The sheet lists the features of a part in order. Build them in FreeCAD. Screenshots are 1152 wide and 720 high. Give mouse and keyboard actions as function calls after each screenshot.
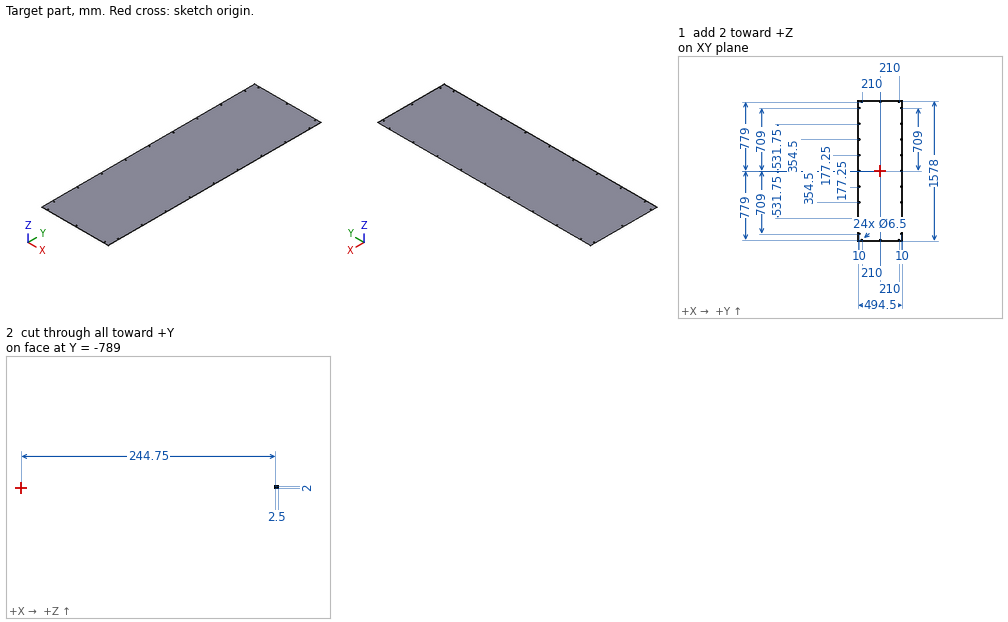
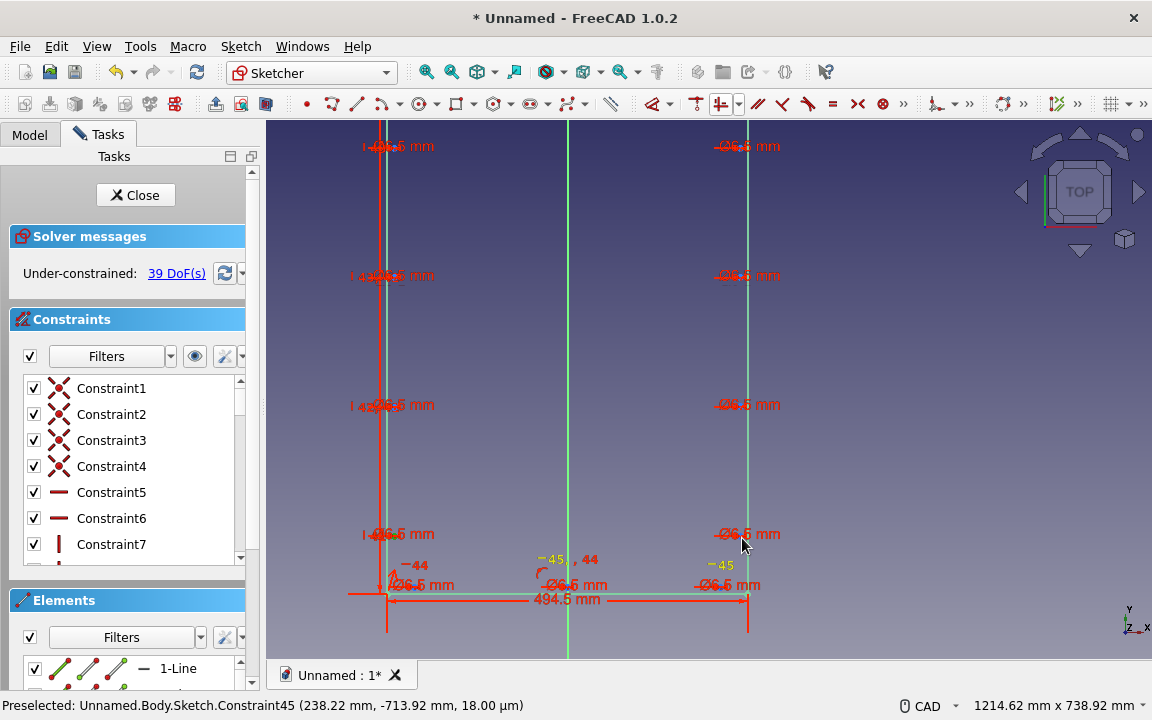
click(741, 536)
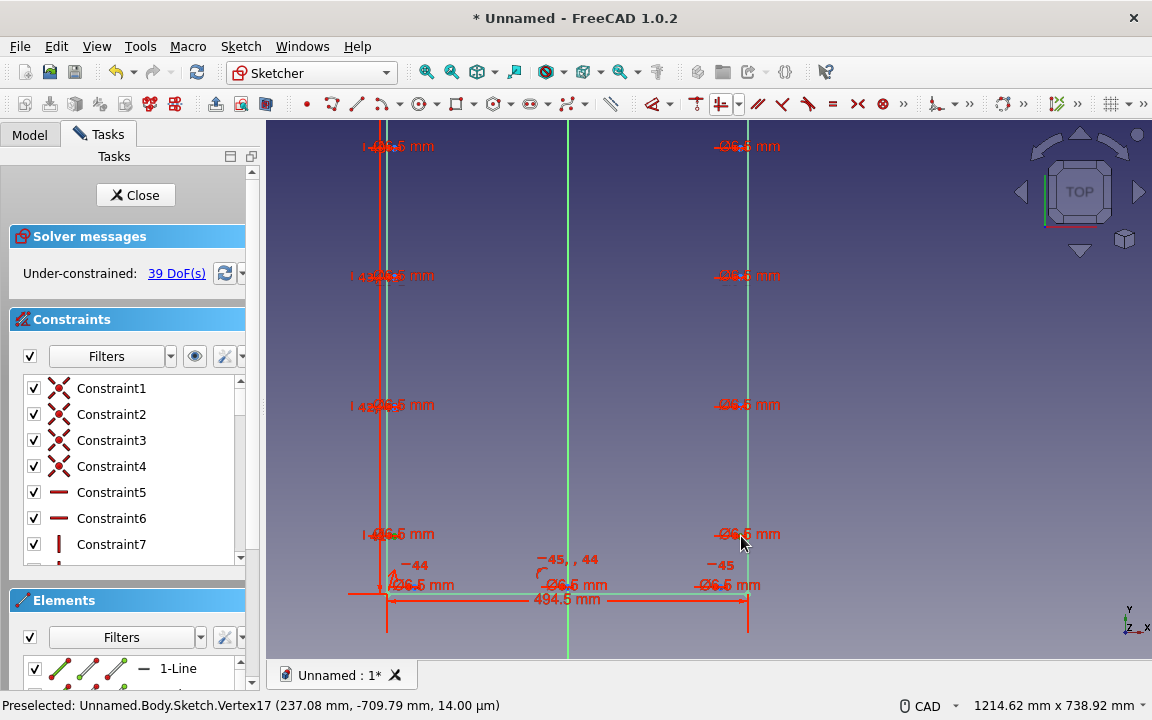
click(738, 104)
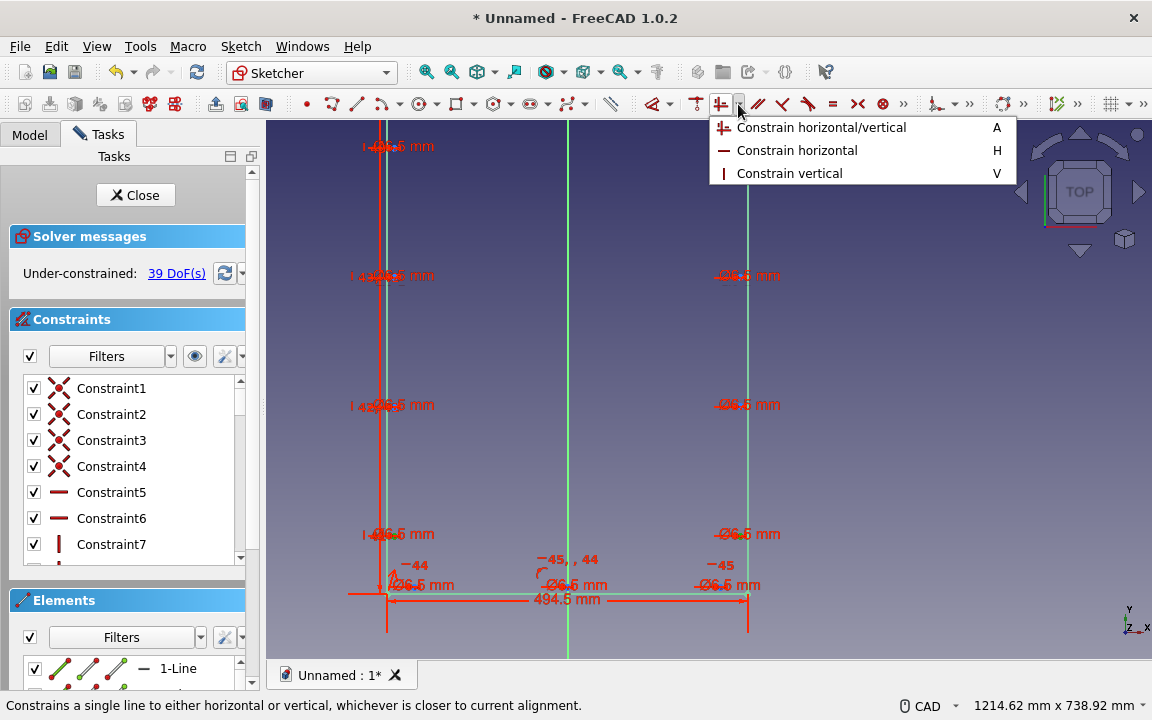
click(863, 150)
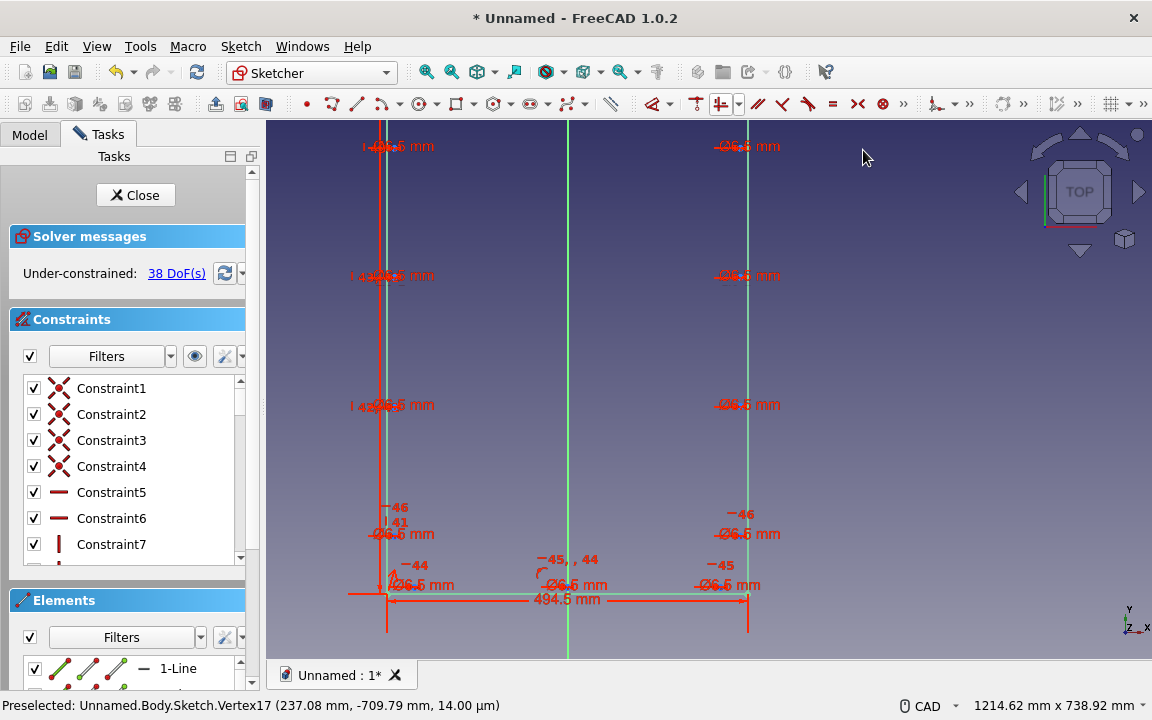
click(741, 536)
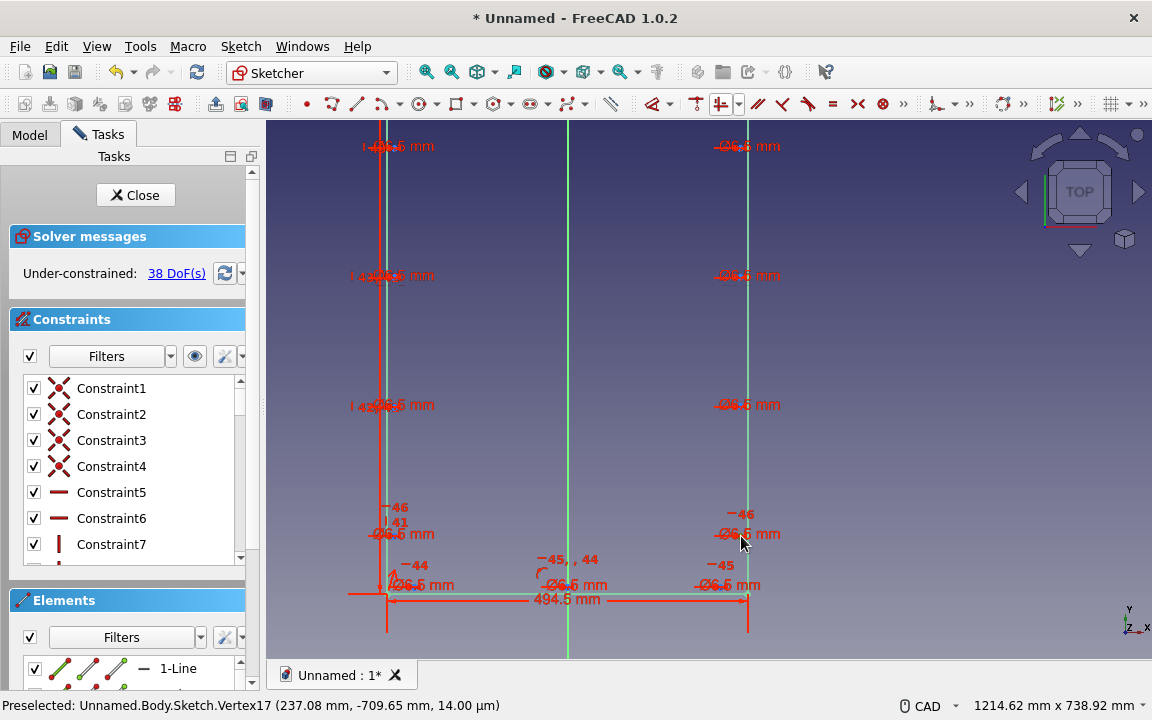
click(740, 407)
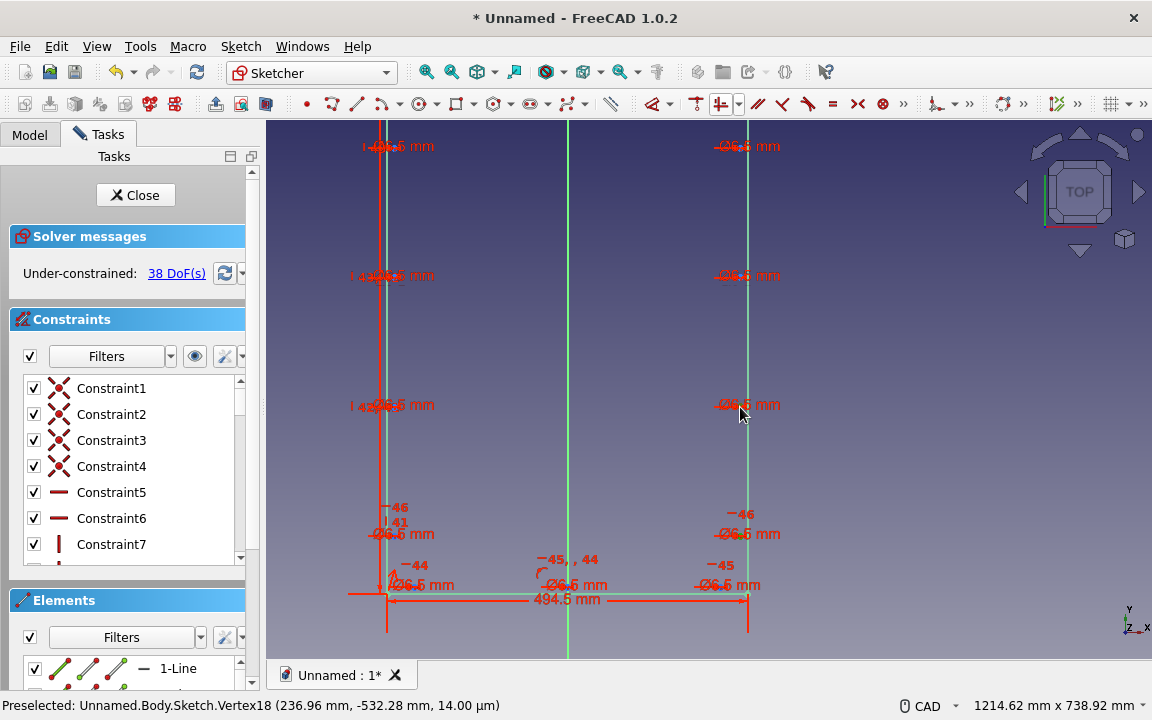
click(738, 104)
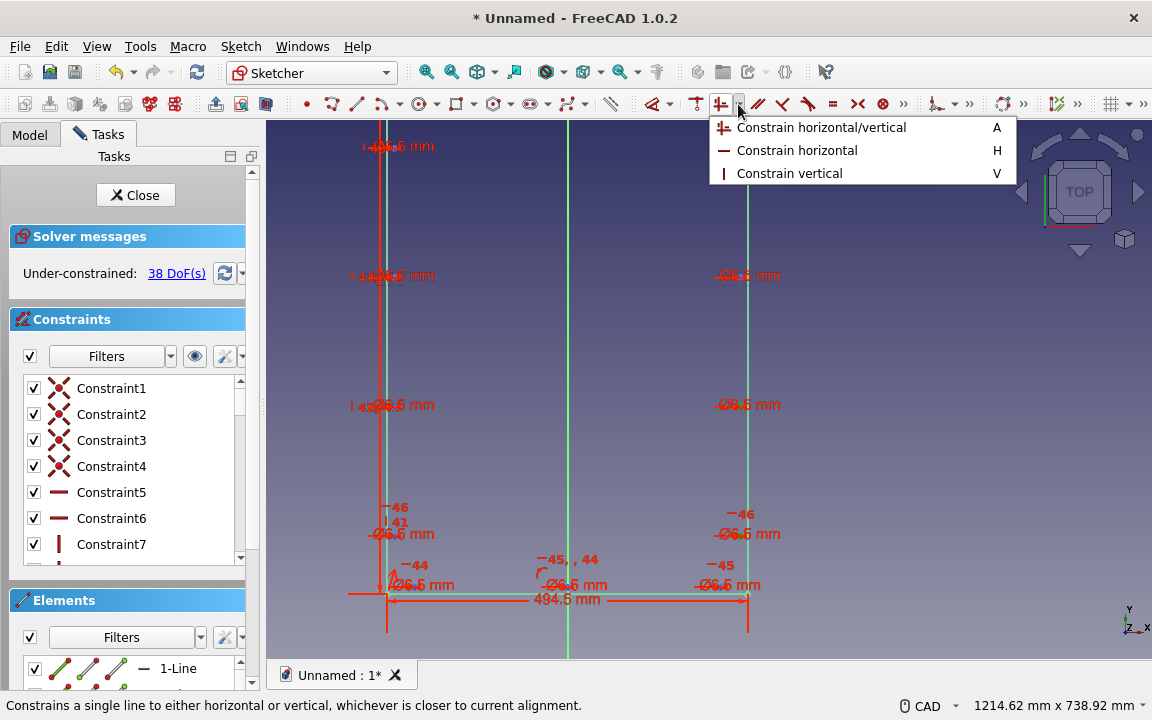
click(863, 174)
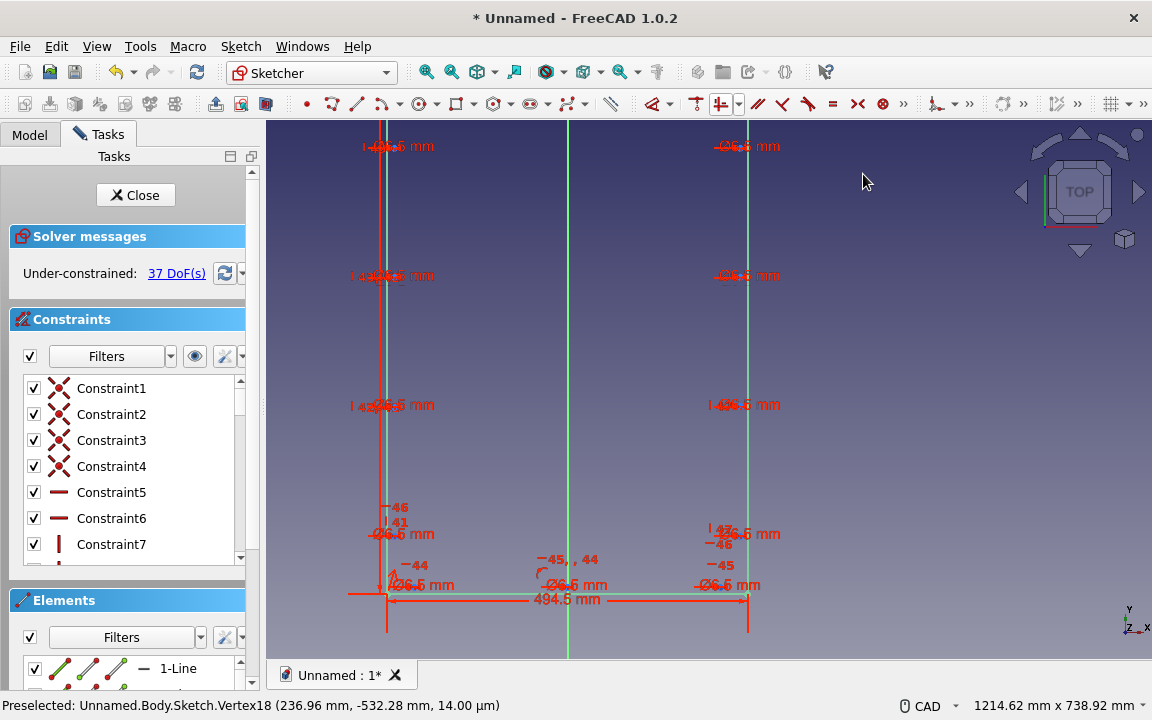
click(394, 407)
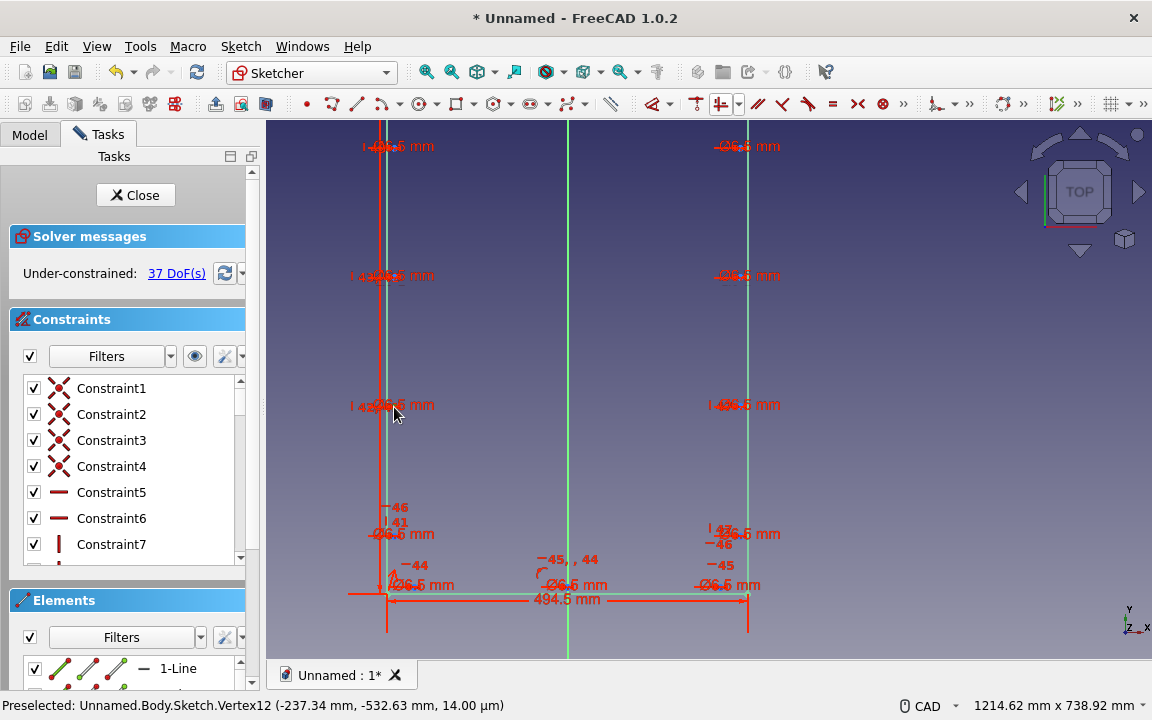
click(741, 407)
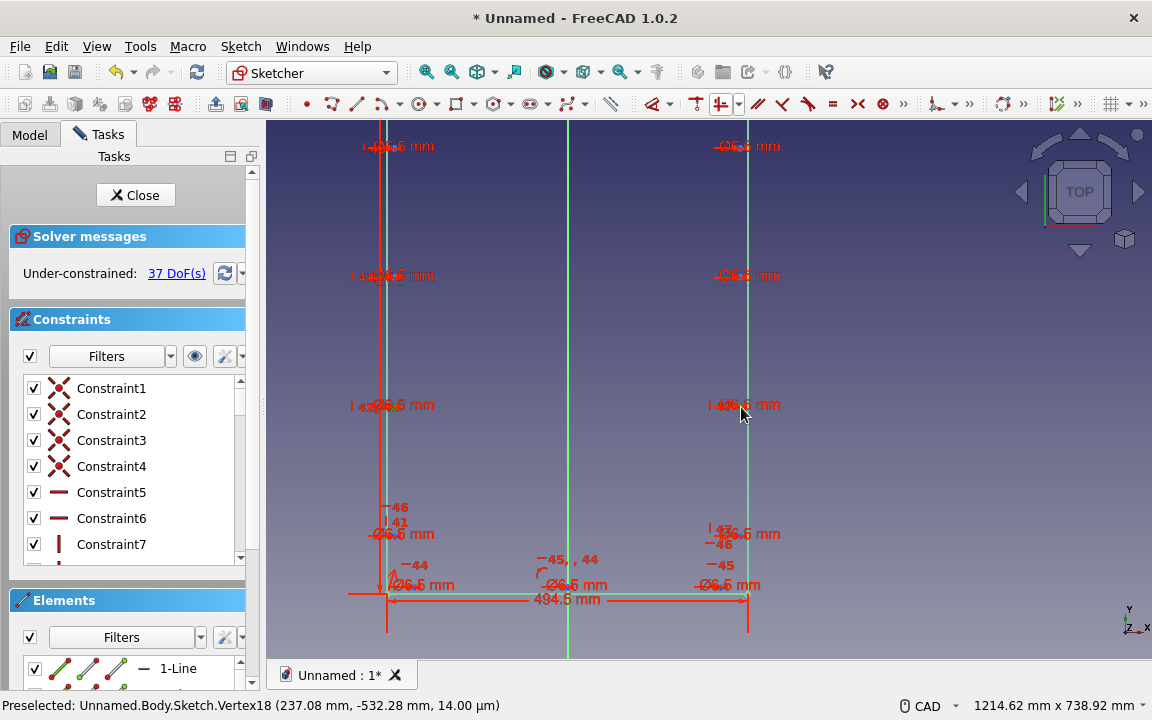
click(738, 104)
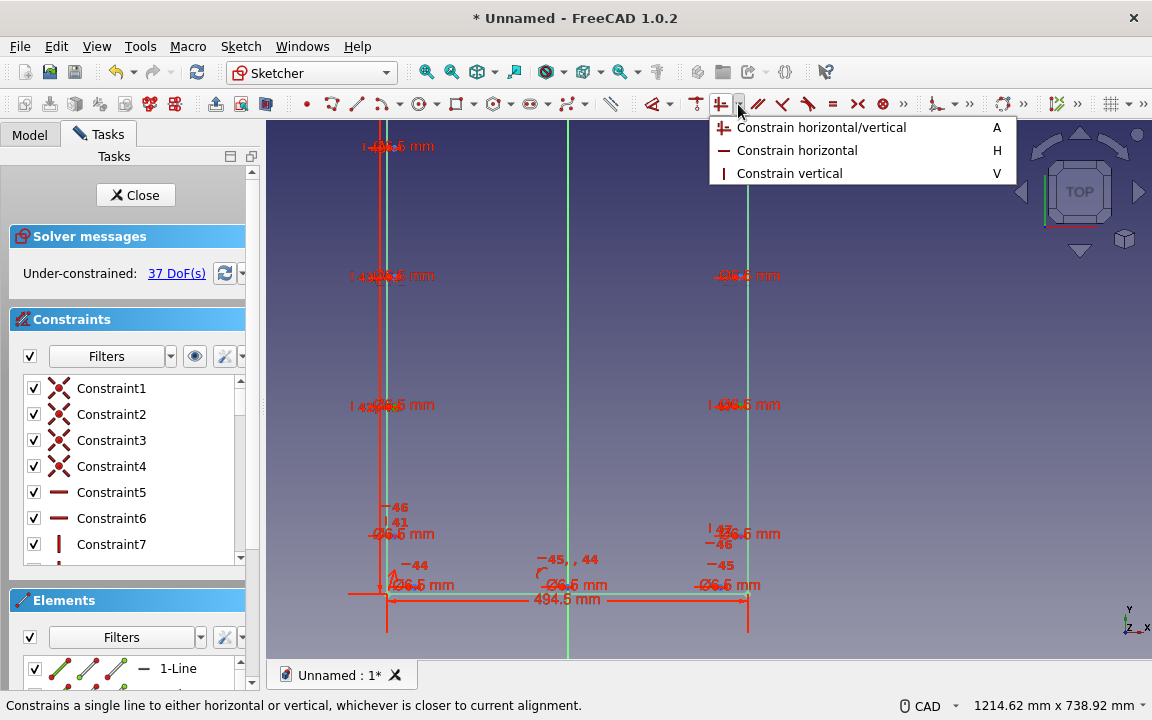
click(863, 150)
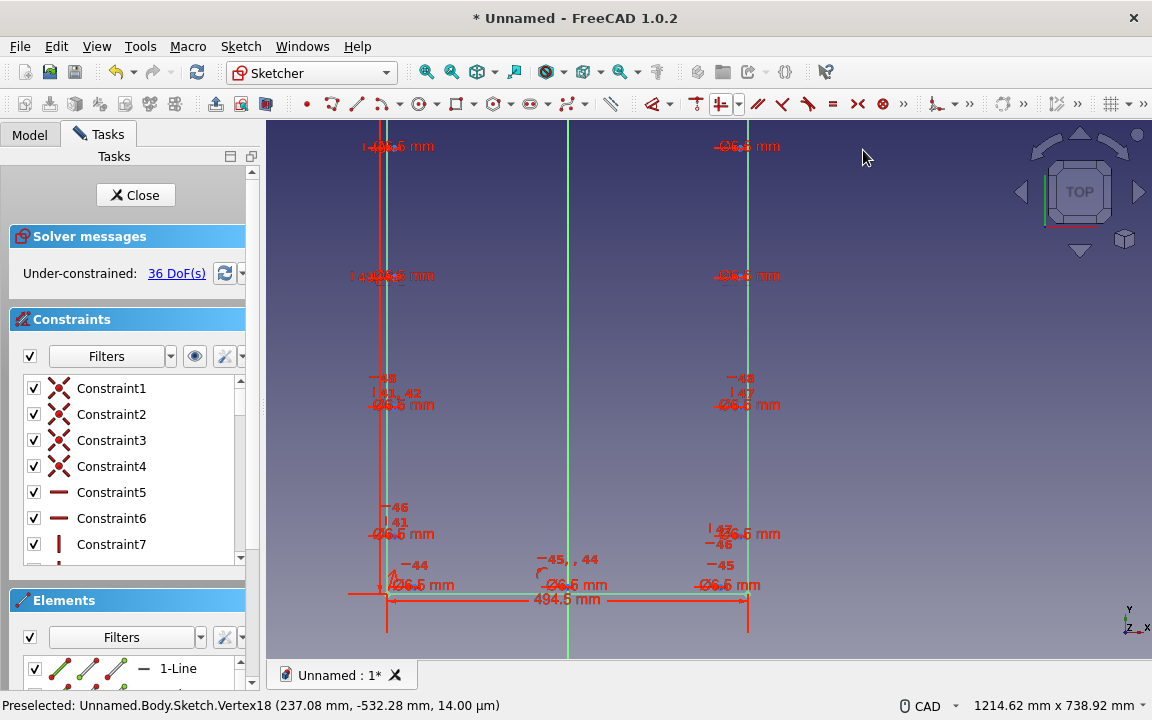
click(741, 407)